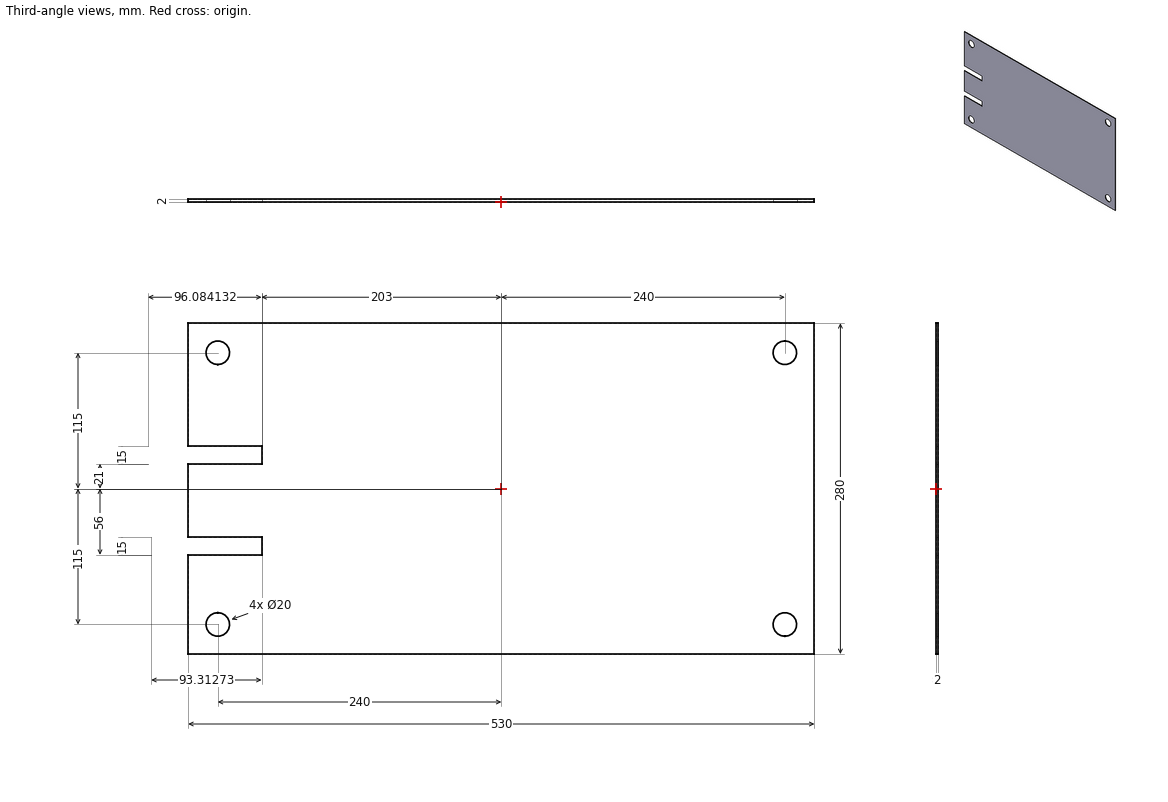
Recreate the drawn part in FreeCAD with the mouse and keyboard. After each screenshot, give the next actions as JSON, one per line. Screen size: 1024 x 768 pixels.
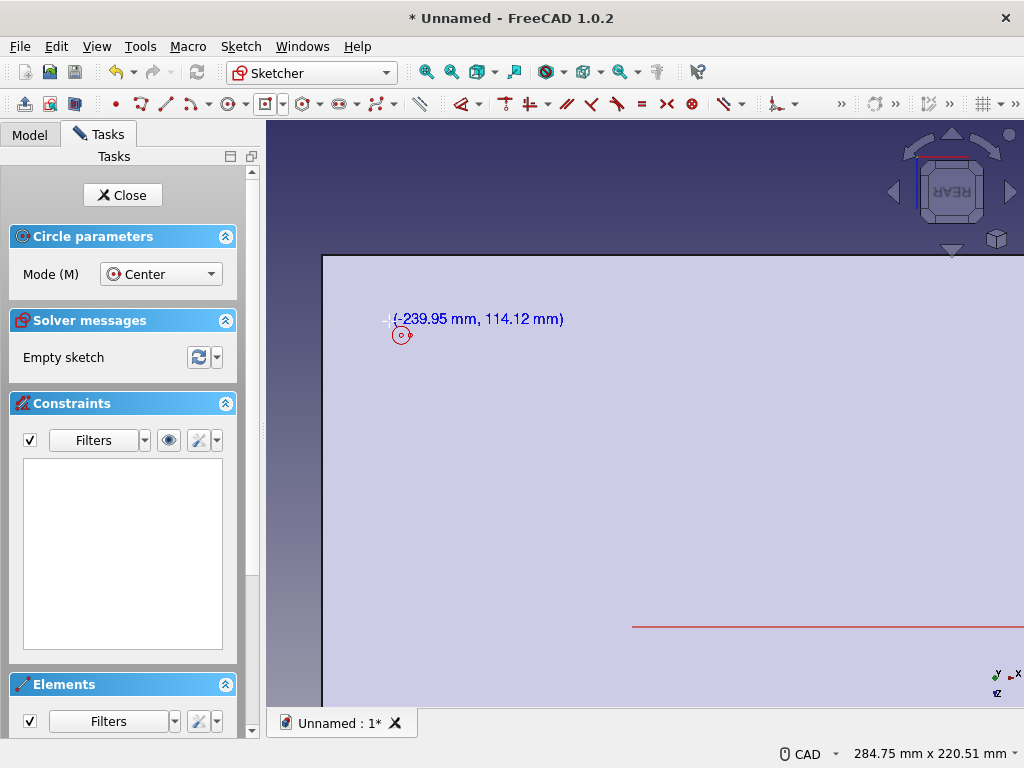
{"action": "left_click", "coordinate": [388, 321]}
{"action": "left_click", "coordinate": [407, 302]}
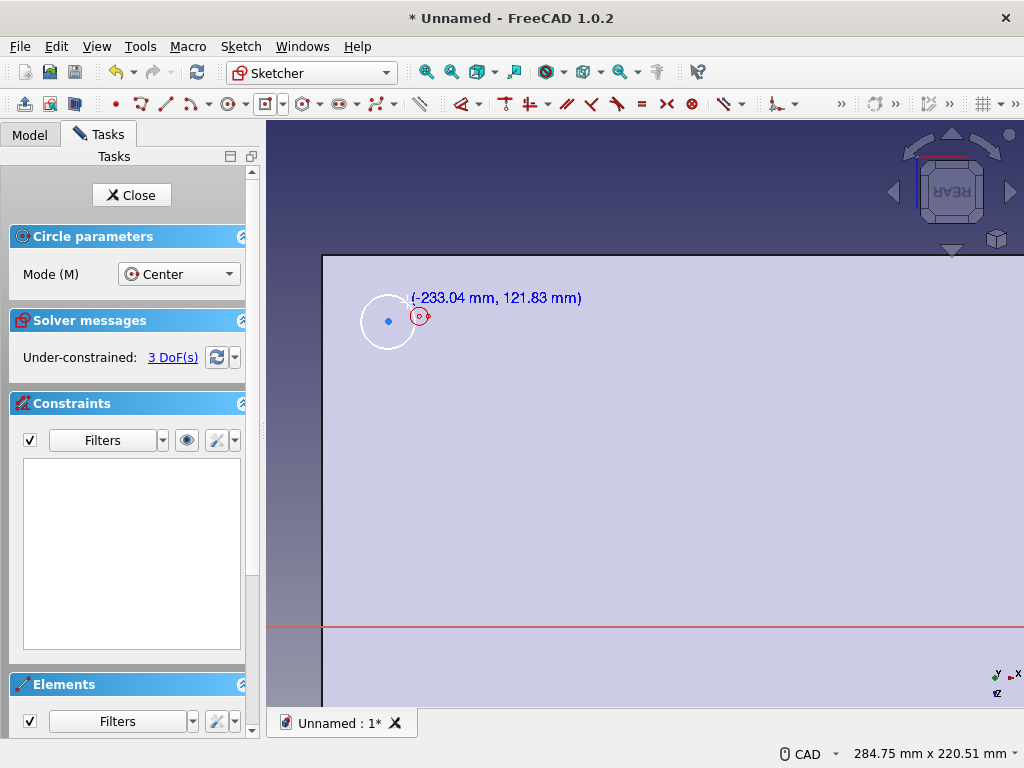
{"action": "scroll", "coordinate": [382, 321], "scroll_direction": "down", "scroll_amount": 6}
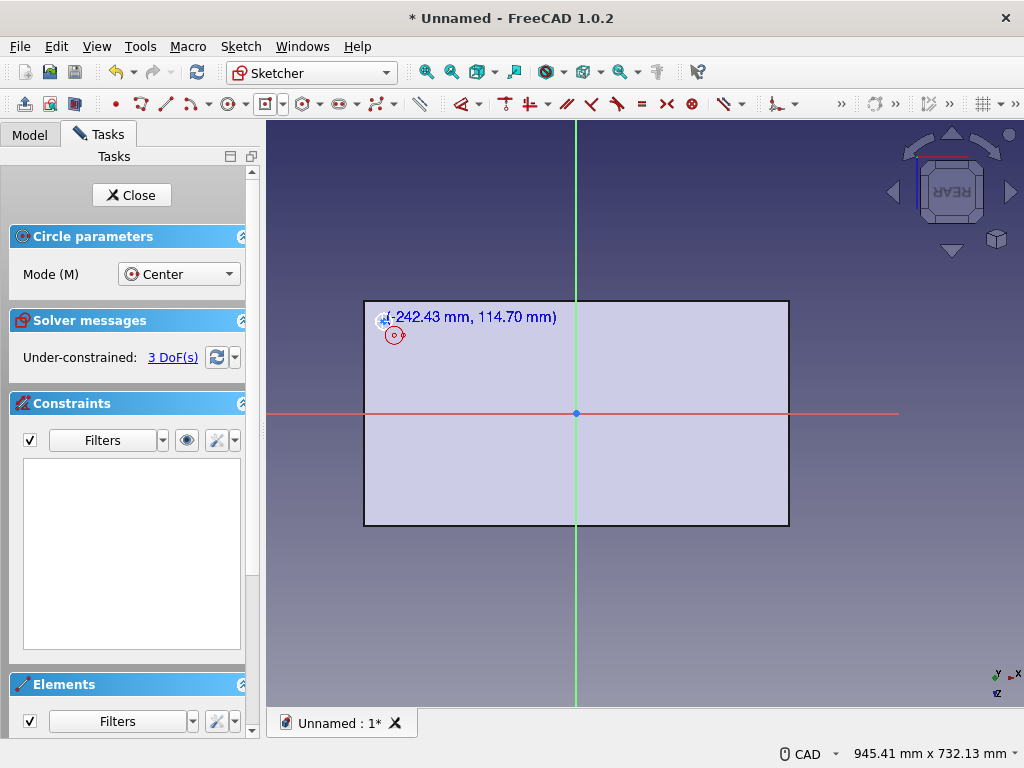
{"action": "scroll", "coordinate": [384, 506], "scroll_direction": "up", "scroll_amount": 6}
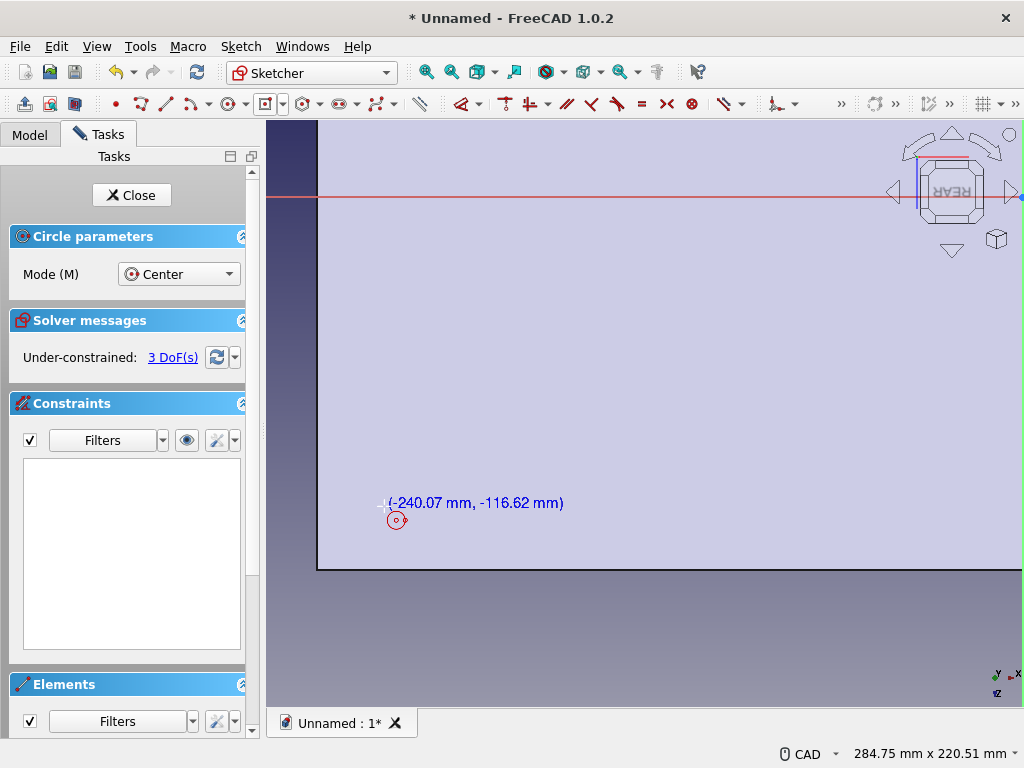
{"action": "left_click", "coordinate": [384, 503]}
{"action": "left_click", "coordinate": [403, 485]}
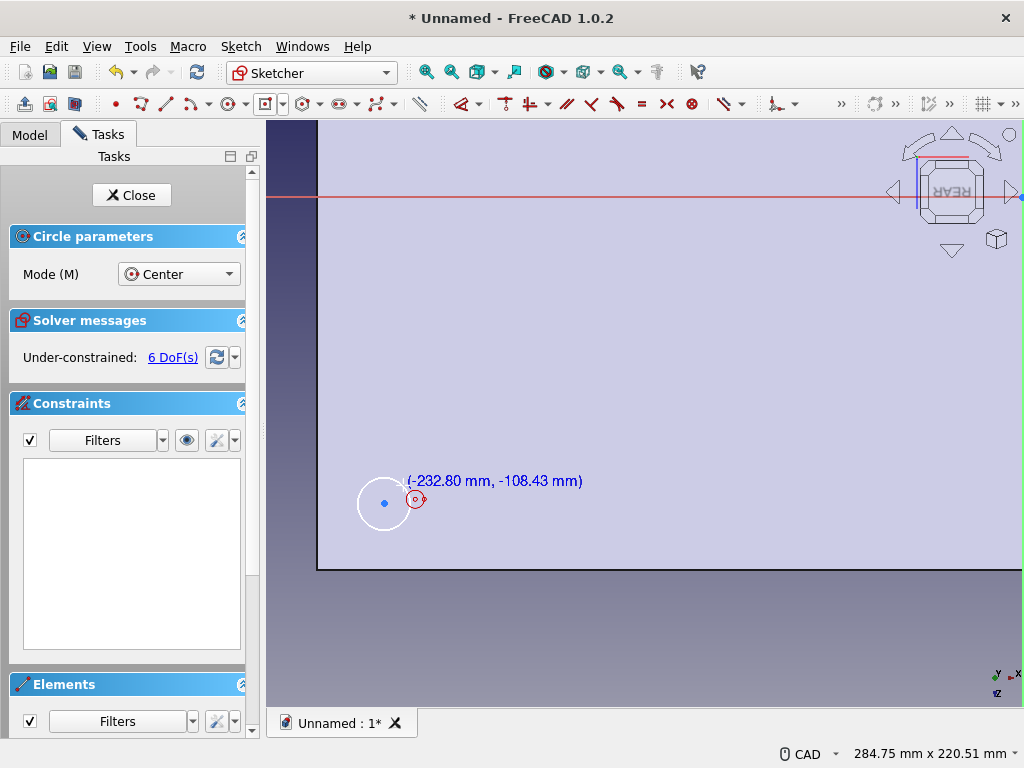
{"action": "scroll", "coordinate": [384, 507], "scroll_direction": "down", "scroll_amount": 6}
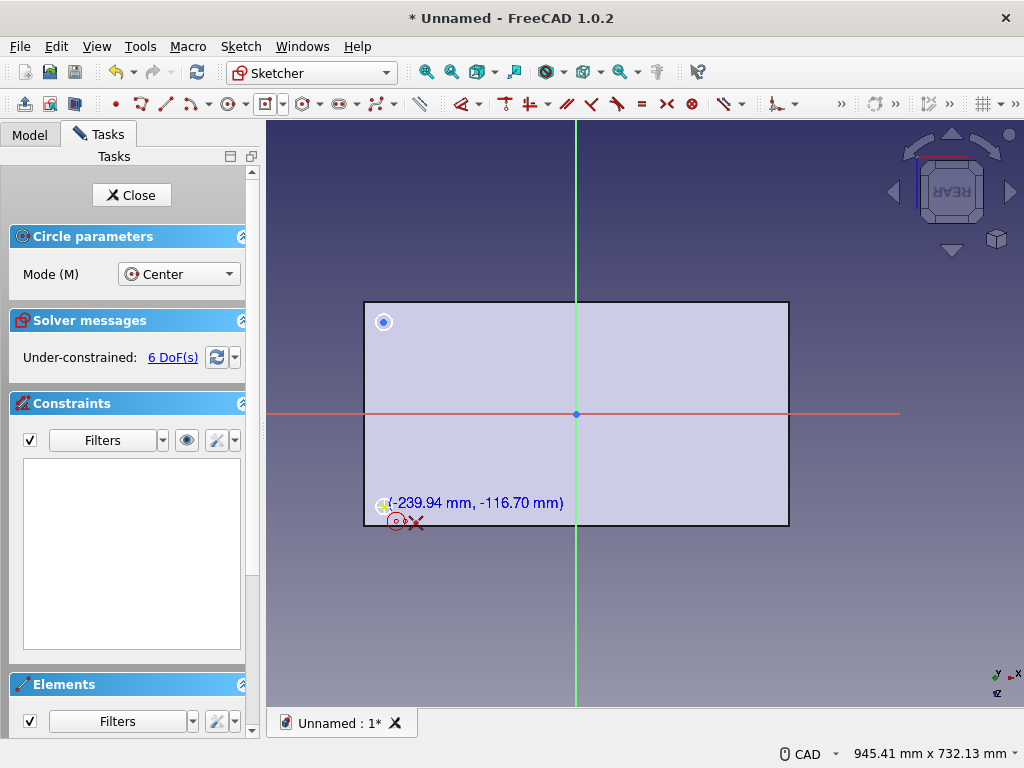
{"action": "scroll", "coordinate": [769, 506], "scroll_direction": "up", "scroll_amount": 6}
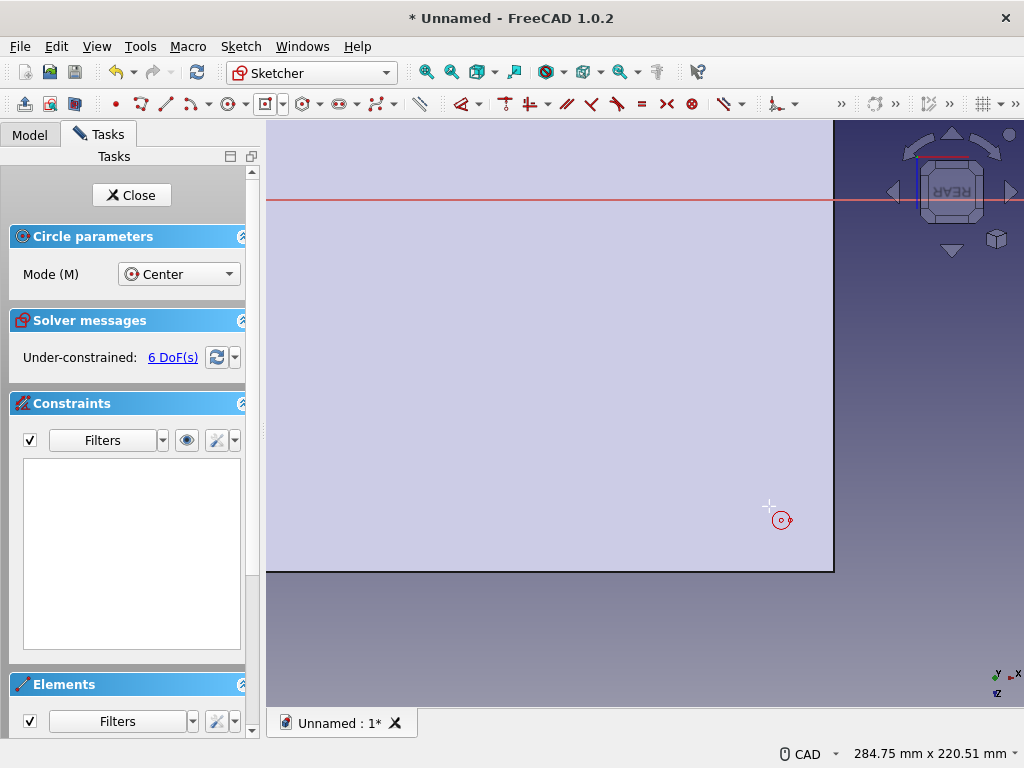
{"action": "left_click", "coordinate": [767, 506]}
{"action": "left_click", "coordinate": [786, 487]}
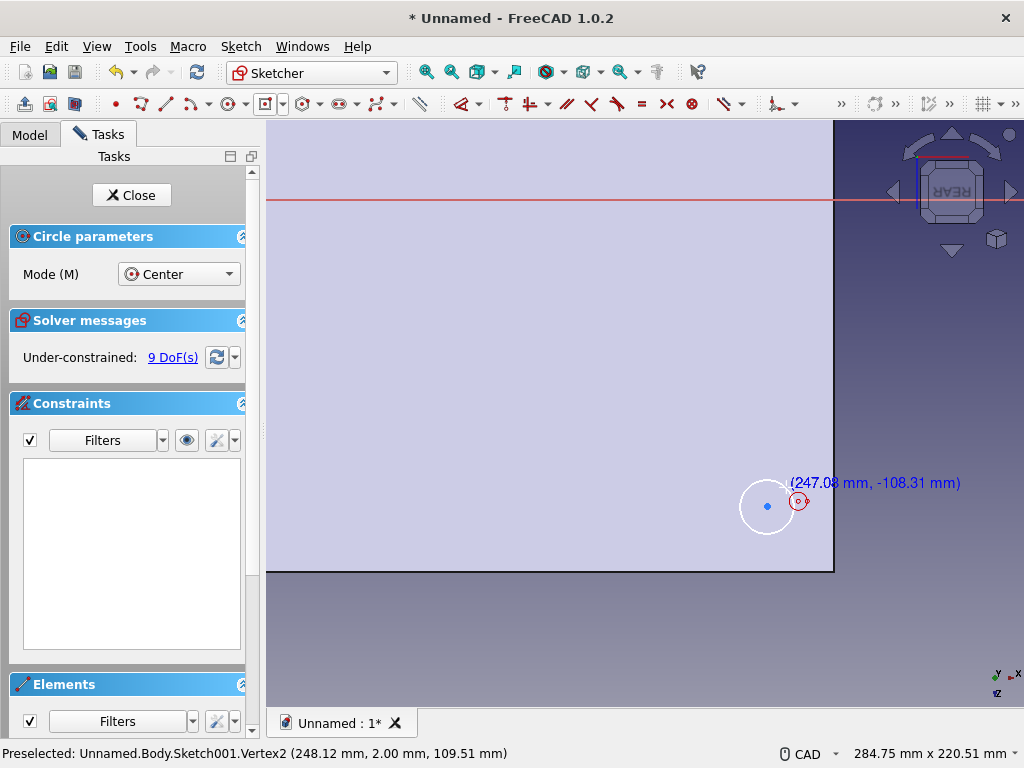
{"action": "scroll", "coordinate": [770, 506], "scroll_direction": "down", "scroll_amount": 6}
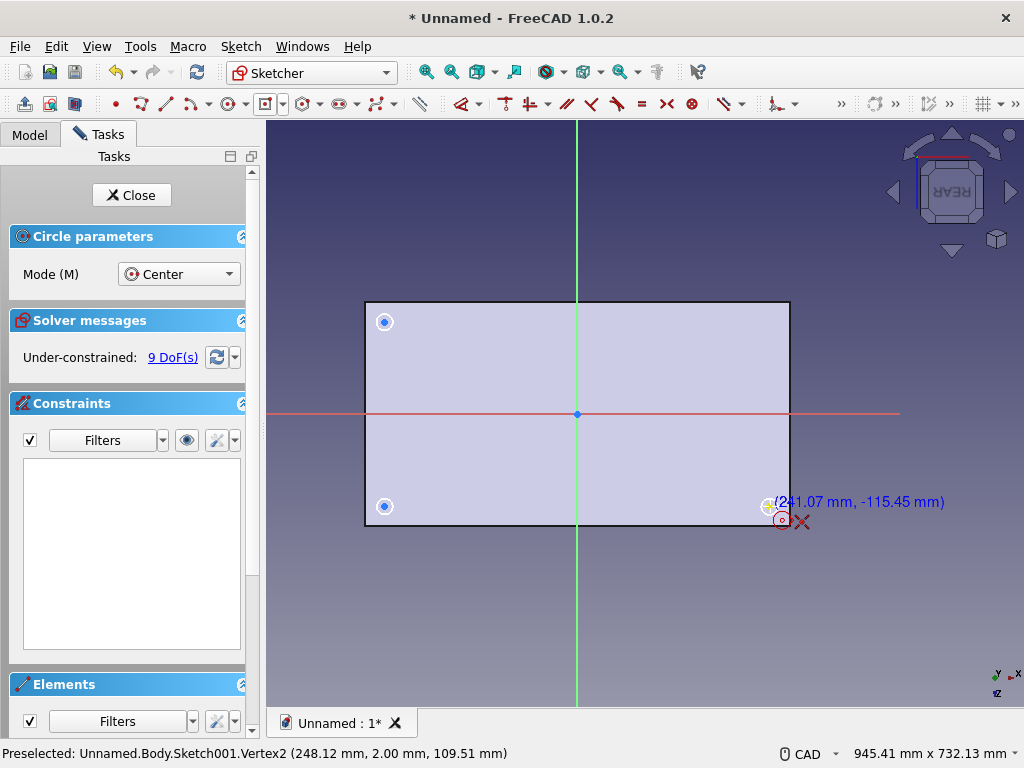
{"action": "scroll", "coordinate": [770, 322], "scroll_direction": "up", "scroll_amount": 6}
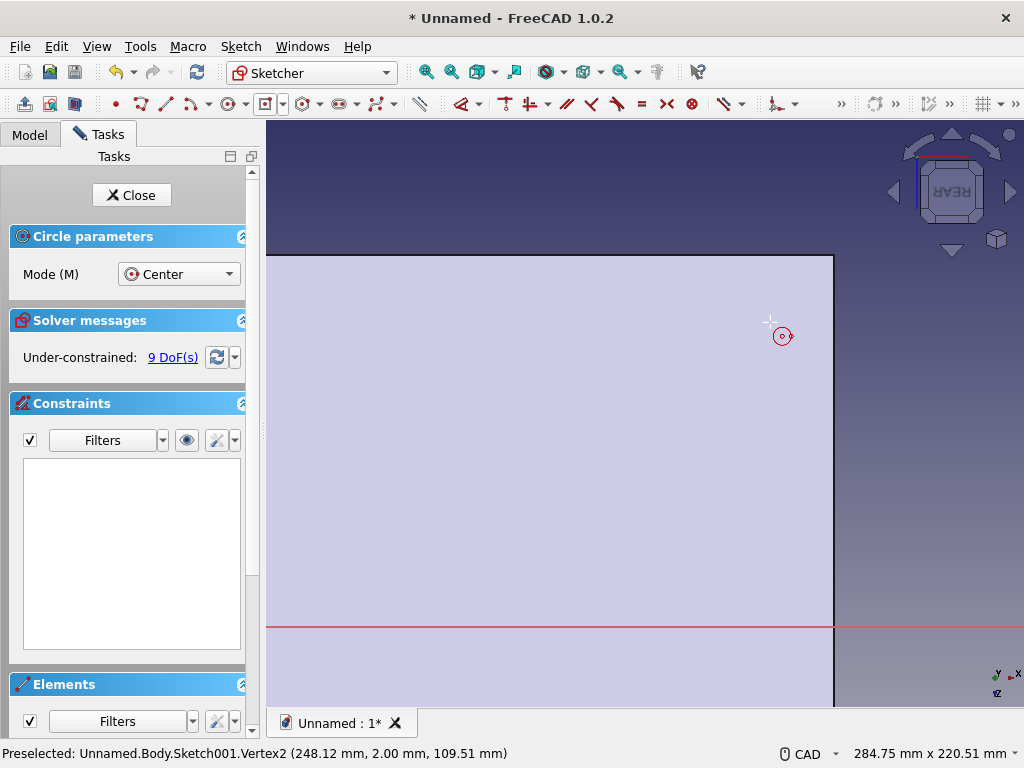
{"action": "left_click", "coordinate": [767, 321]}
{"action": "left_click", "coordinate": [786, 302]}
{"action": "key", "text": "Escape"}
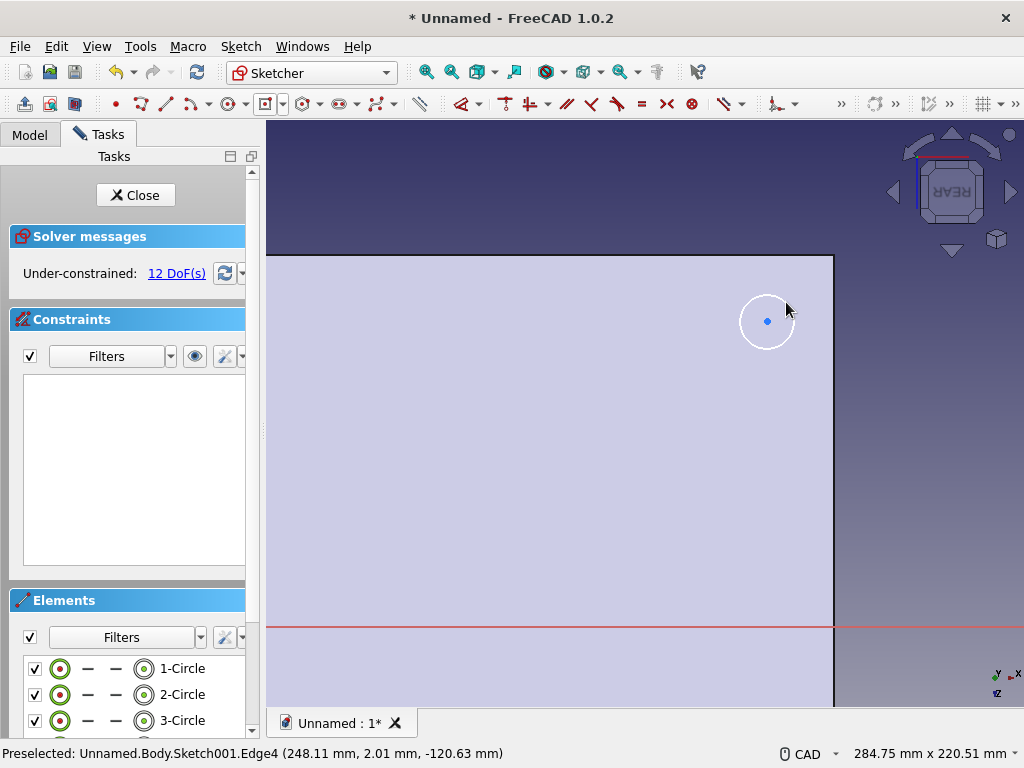
{"action": "scroll", "coordinate": [770, 321], "scroll_direction": "down", "scroll_amount": 6}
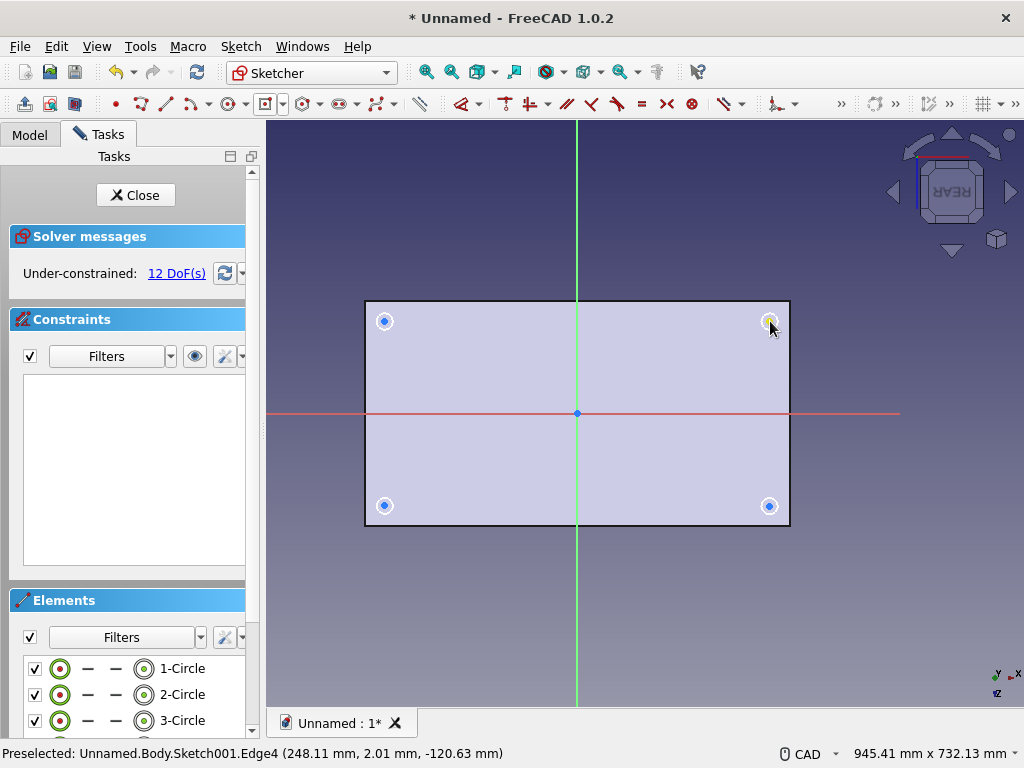
{"action": "scroll", "coordinate": [390, 316], "scroll_direction": "up", "scroll_amount": 3}